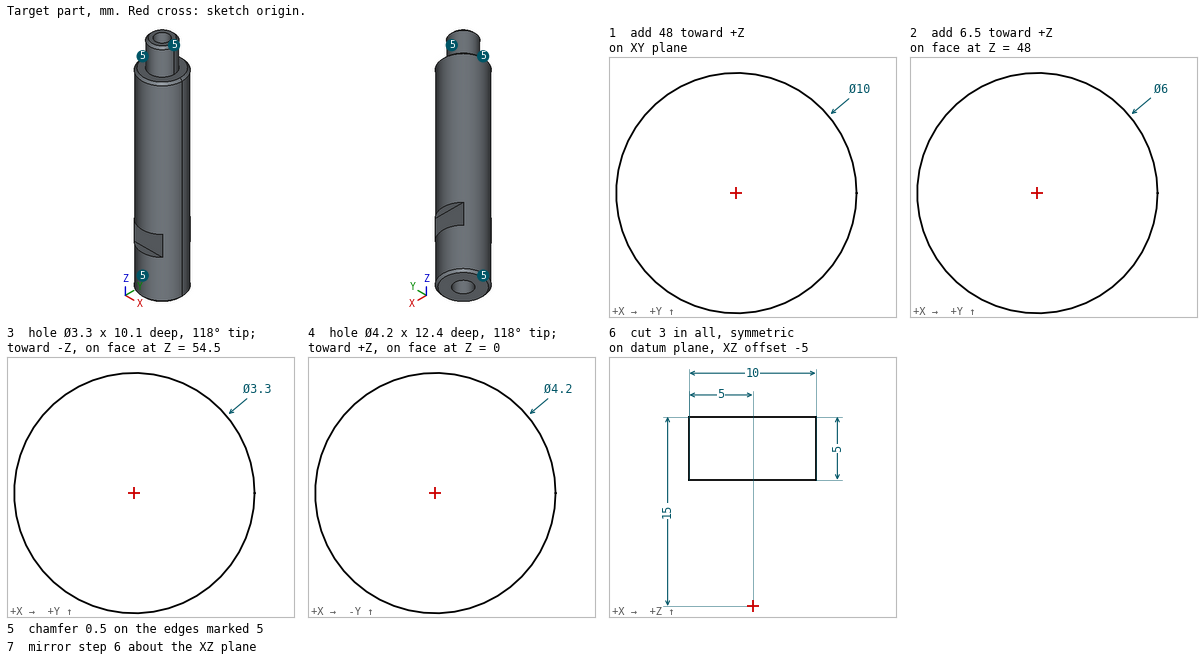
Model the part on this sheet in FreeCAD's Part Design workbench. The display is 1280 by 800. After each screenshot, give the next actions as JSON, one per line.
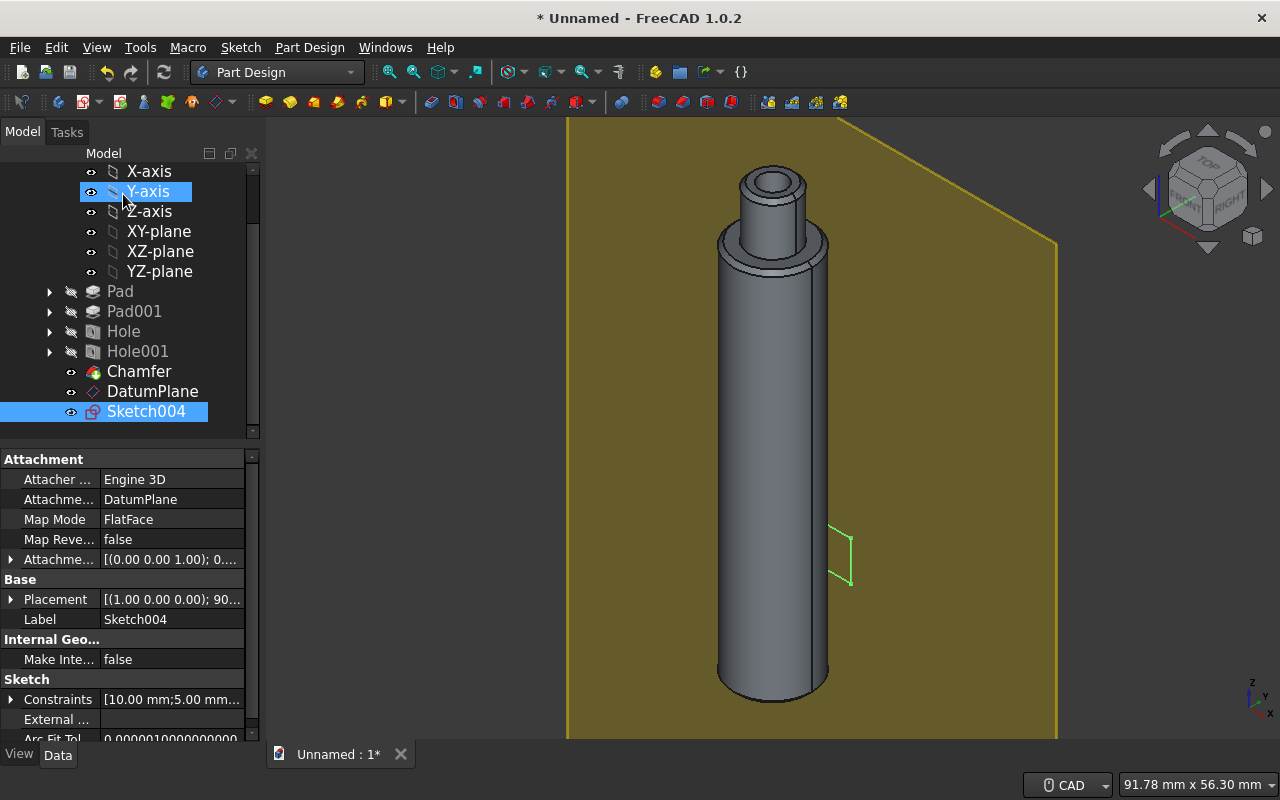
{"action": "left_click", "coordinate": [432, 102]}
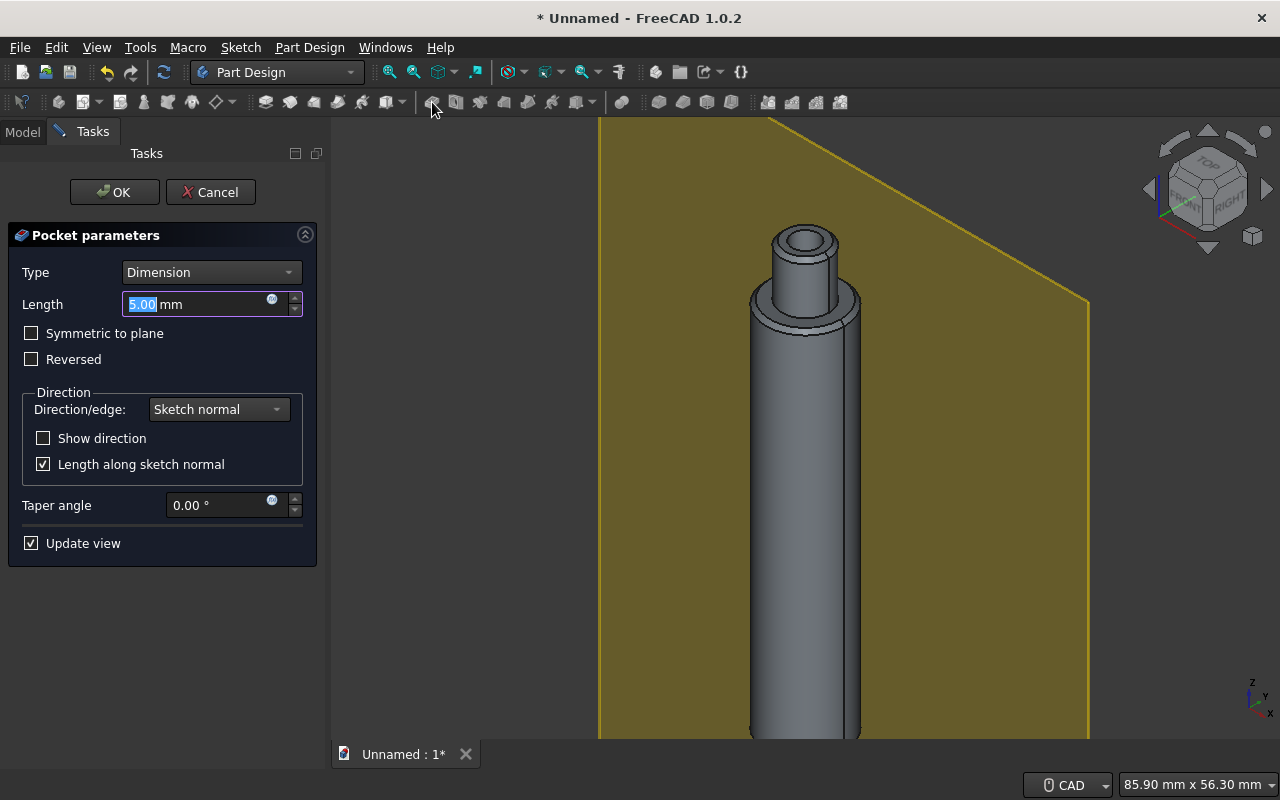
{"action": "type", "text": "3"}
{"action": "key", "text": "Tab"}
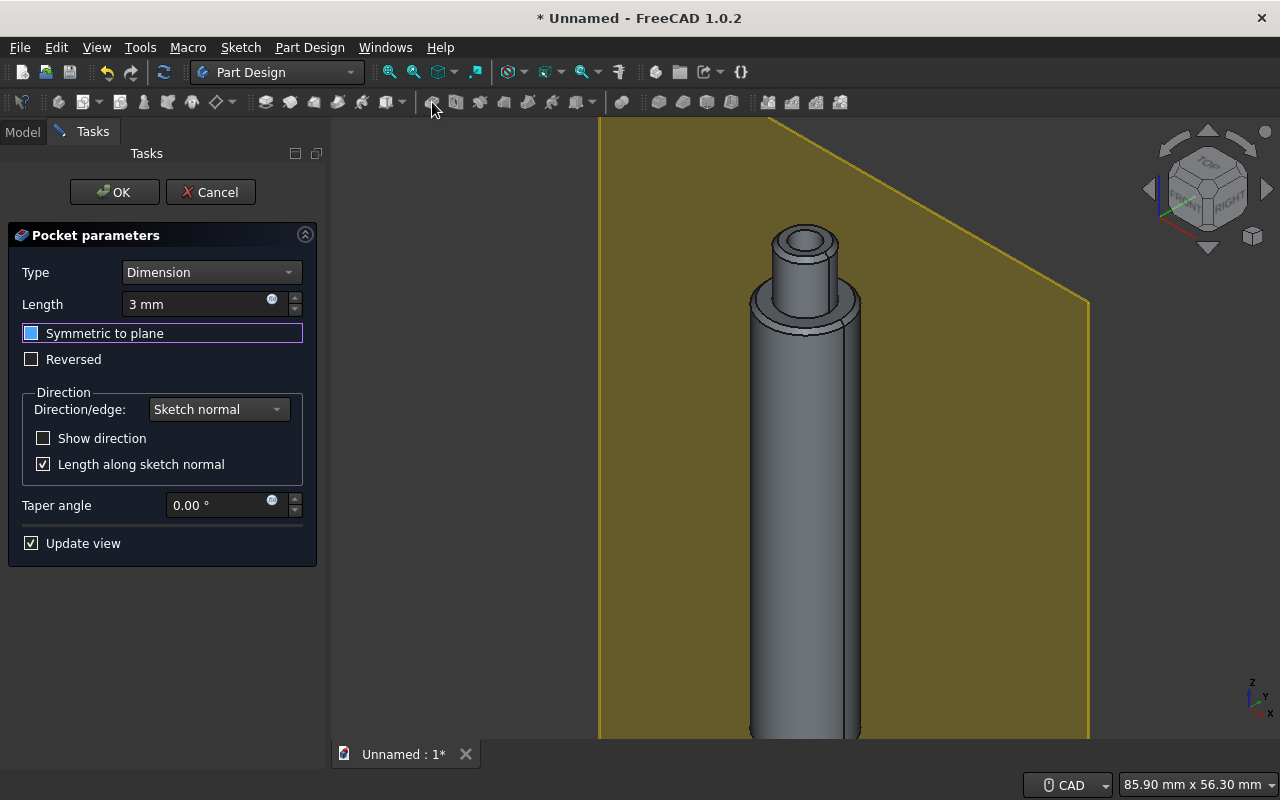
{"action": "left_click", "coordinate": [30, 333]}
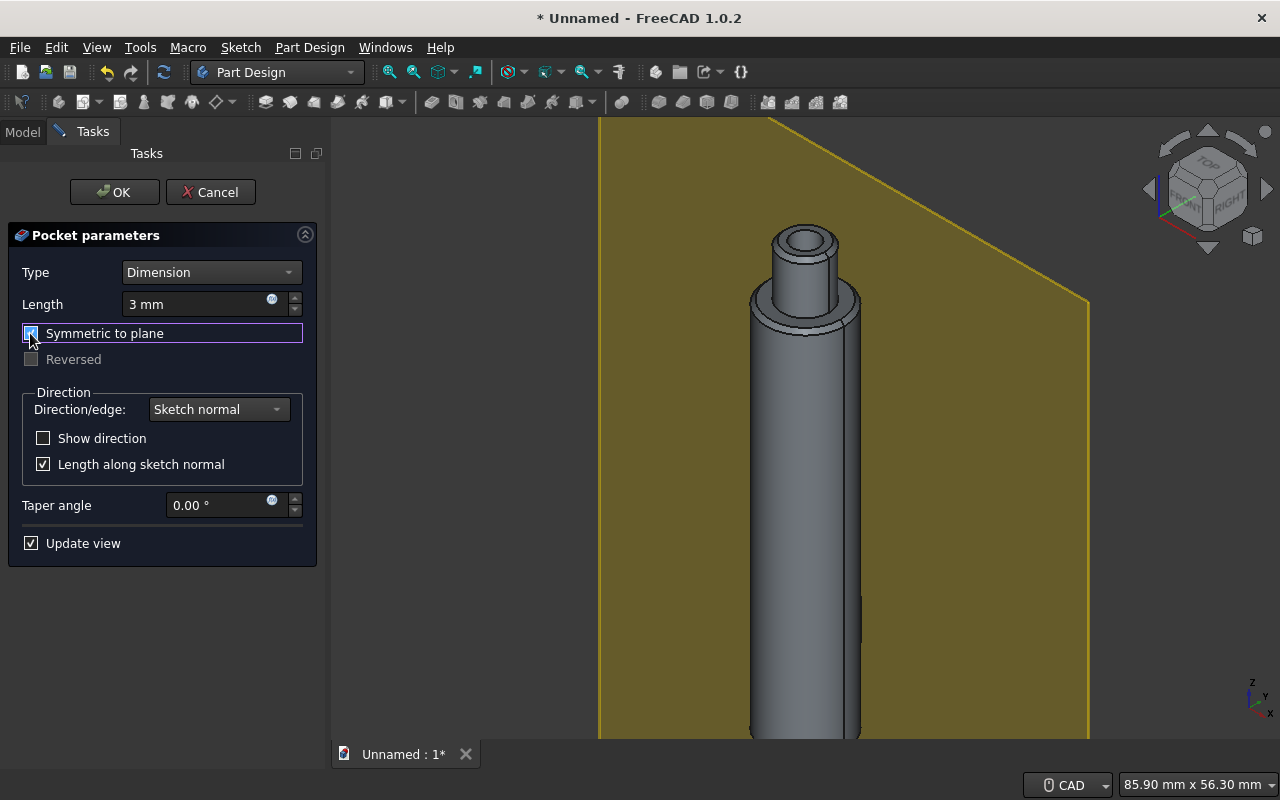
{"action": "left_click", "coordinate": [115, 192]}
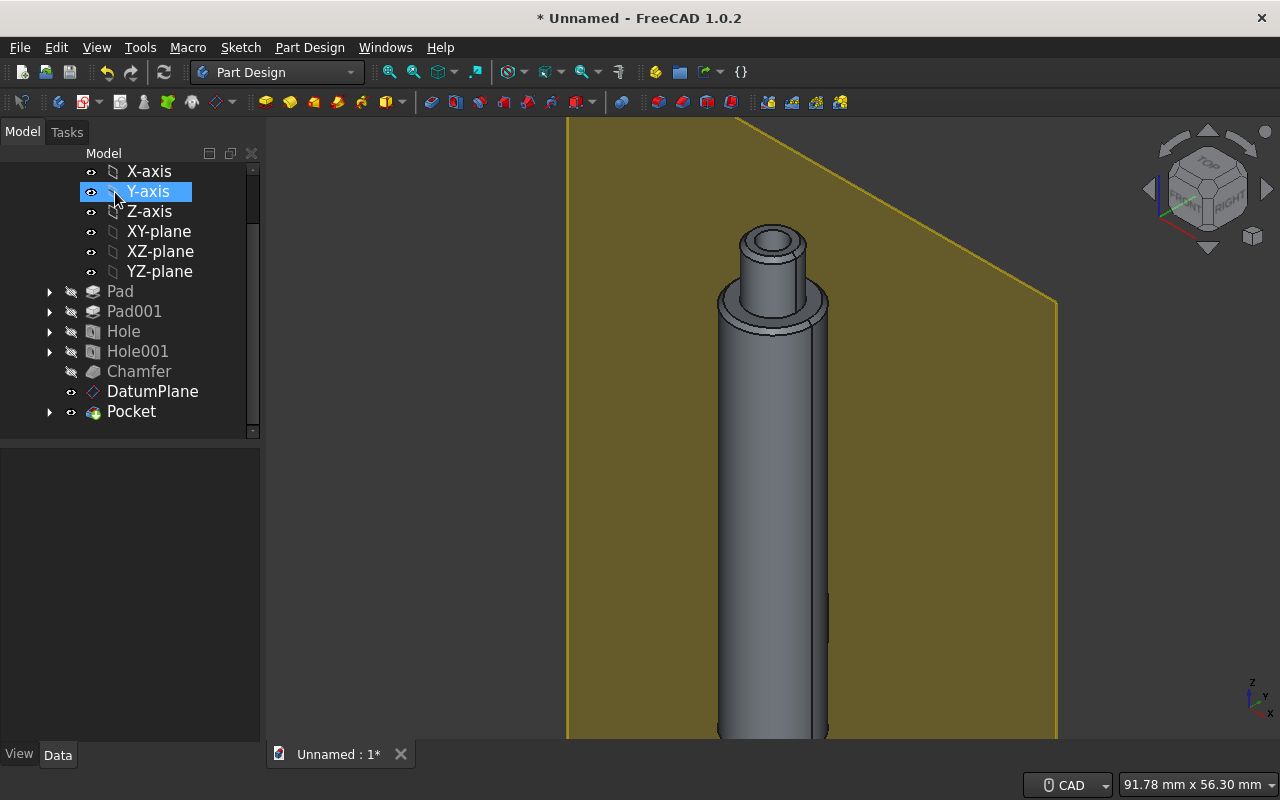
{"action": "left_click", "coordinate": [116, 392]}
{"action": "key", "text": "space"}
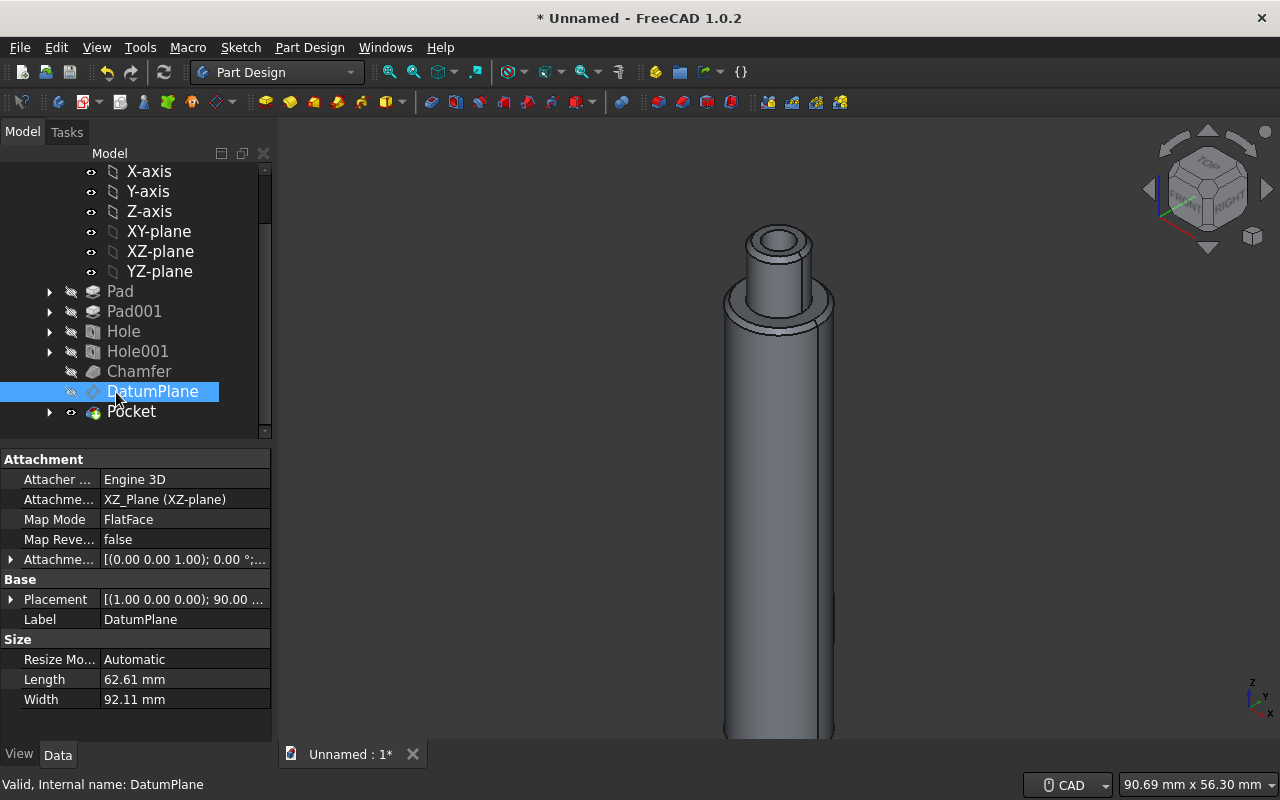
{"action": "left_click", "coordinate": [390, 72]}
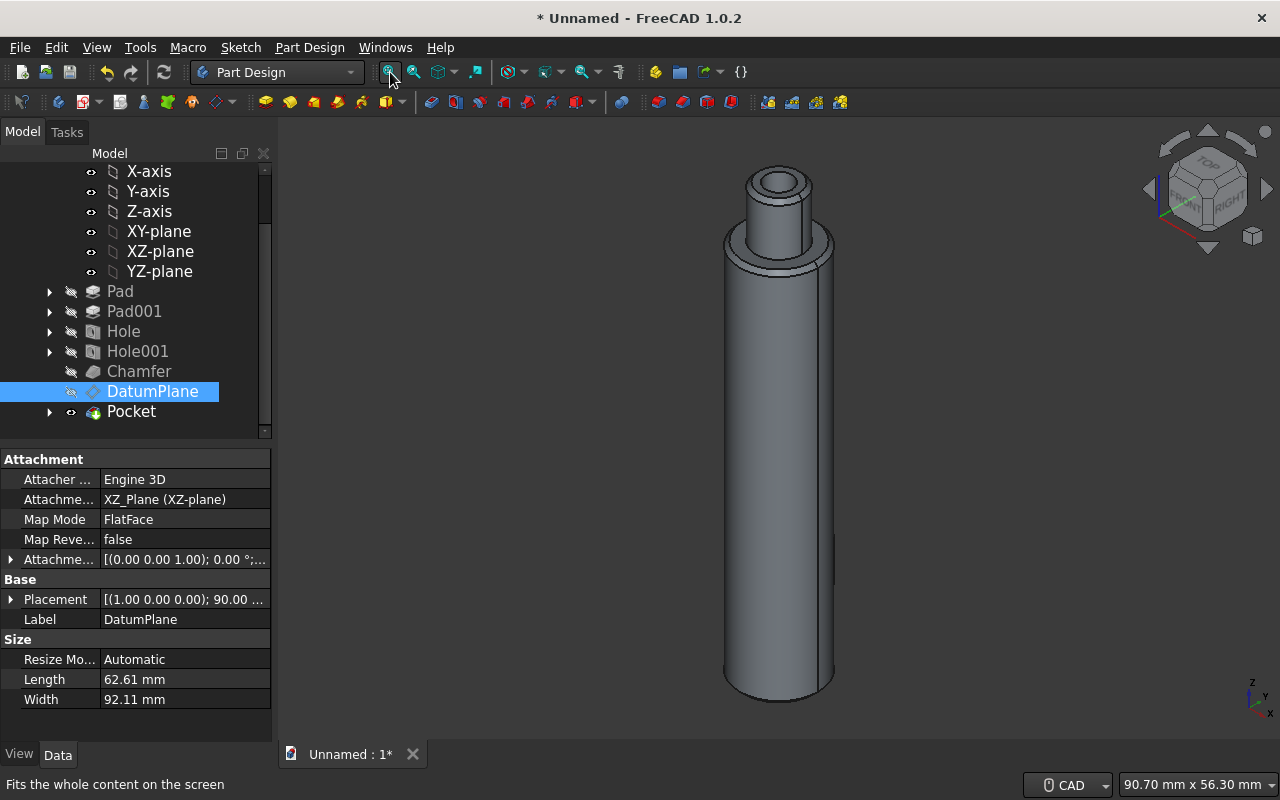
{"action": "left_click", "coordinate": [116, 412]}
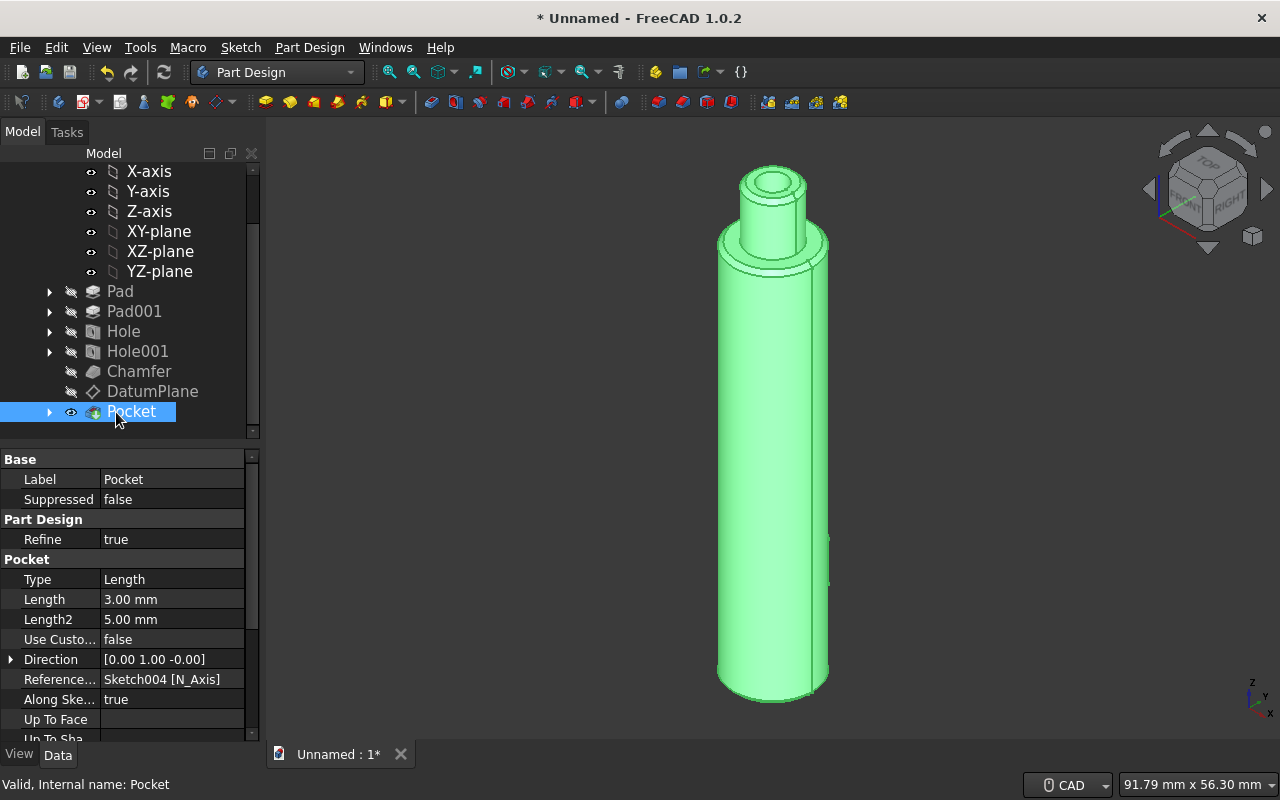
{"action": "left_click", "coordinate": [768, 102]}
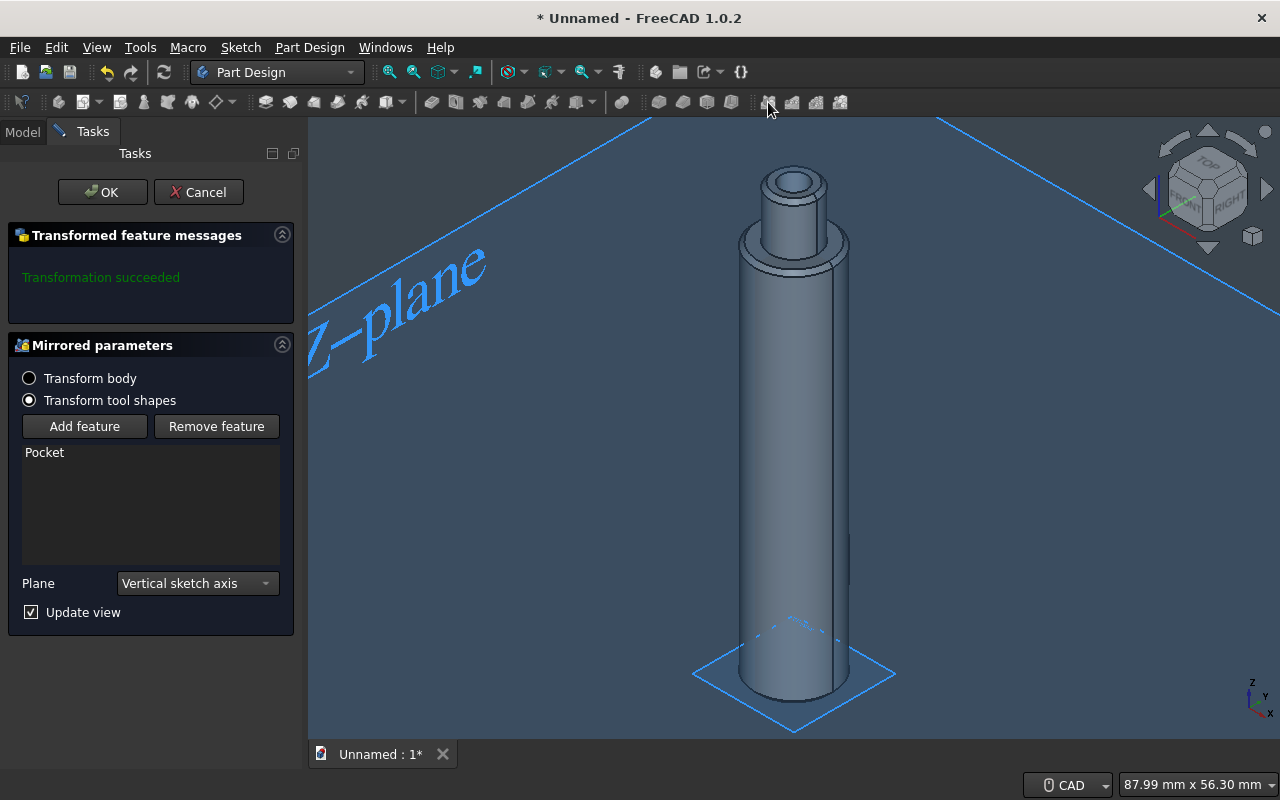
{"action": "left_click", "coordinate": [198, 584]}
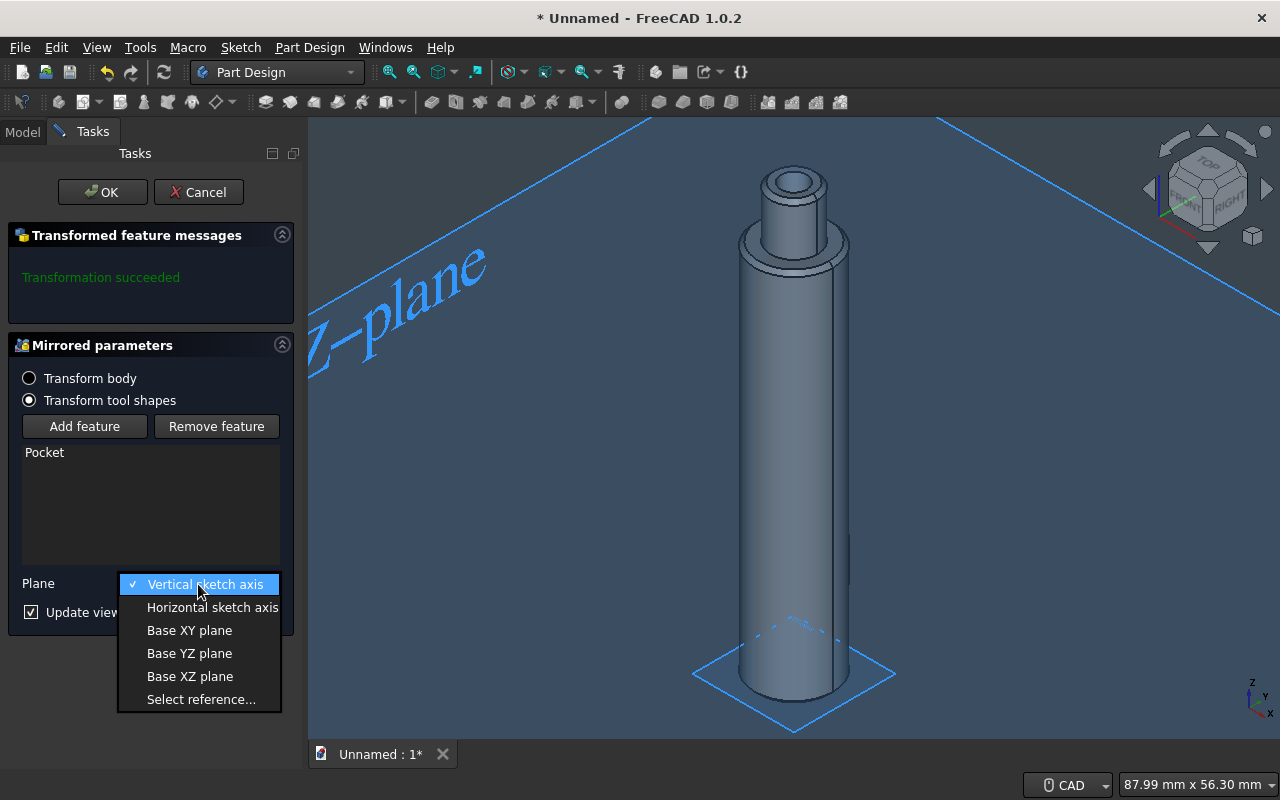
{"action": "left_click", "coordinate": [198, 676]}